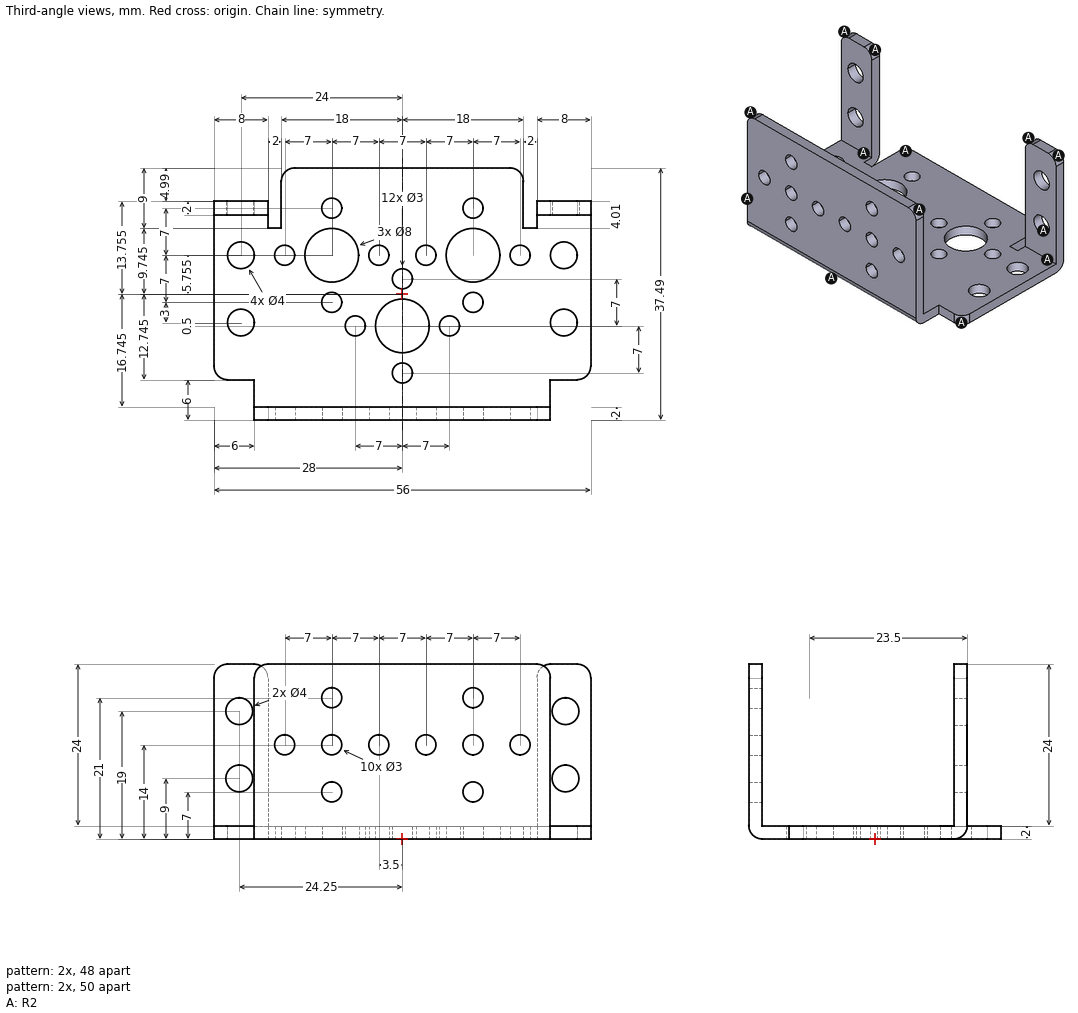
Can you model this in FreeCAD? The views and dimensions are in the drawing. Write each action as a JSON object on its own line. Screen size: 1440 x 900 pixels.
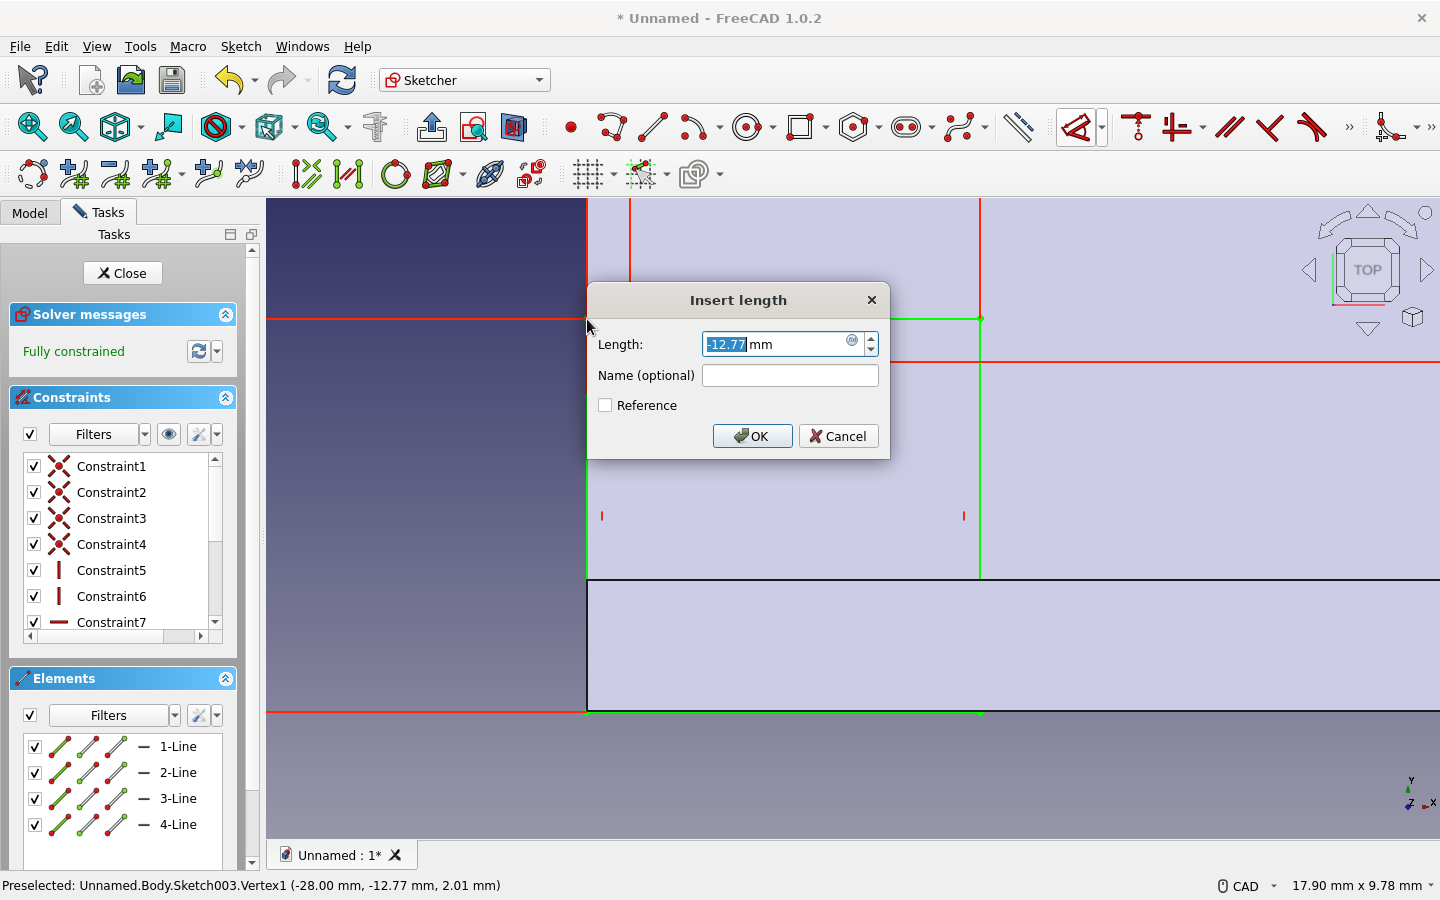
{"action": "type", "text": "-12.745"}
{"action": "key", "text": "Return"}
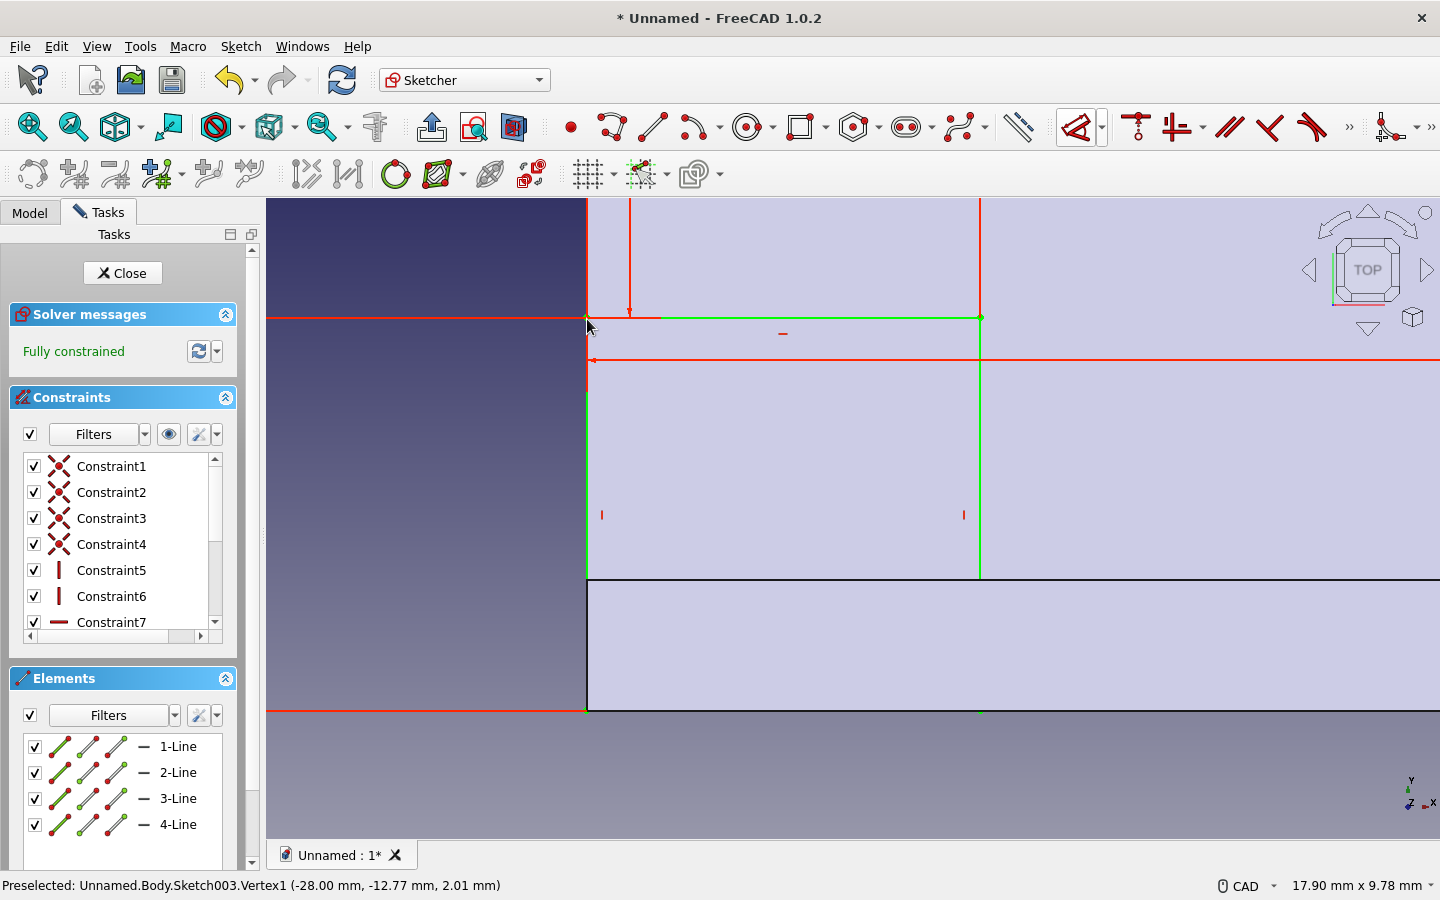
{"action": "left_click", "coordinate": [123, 273]}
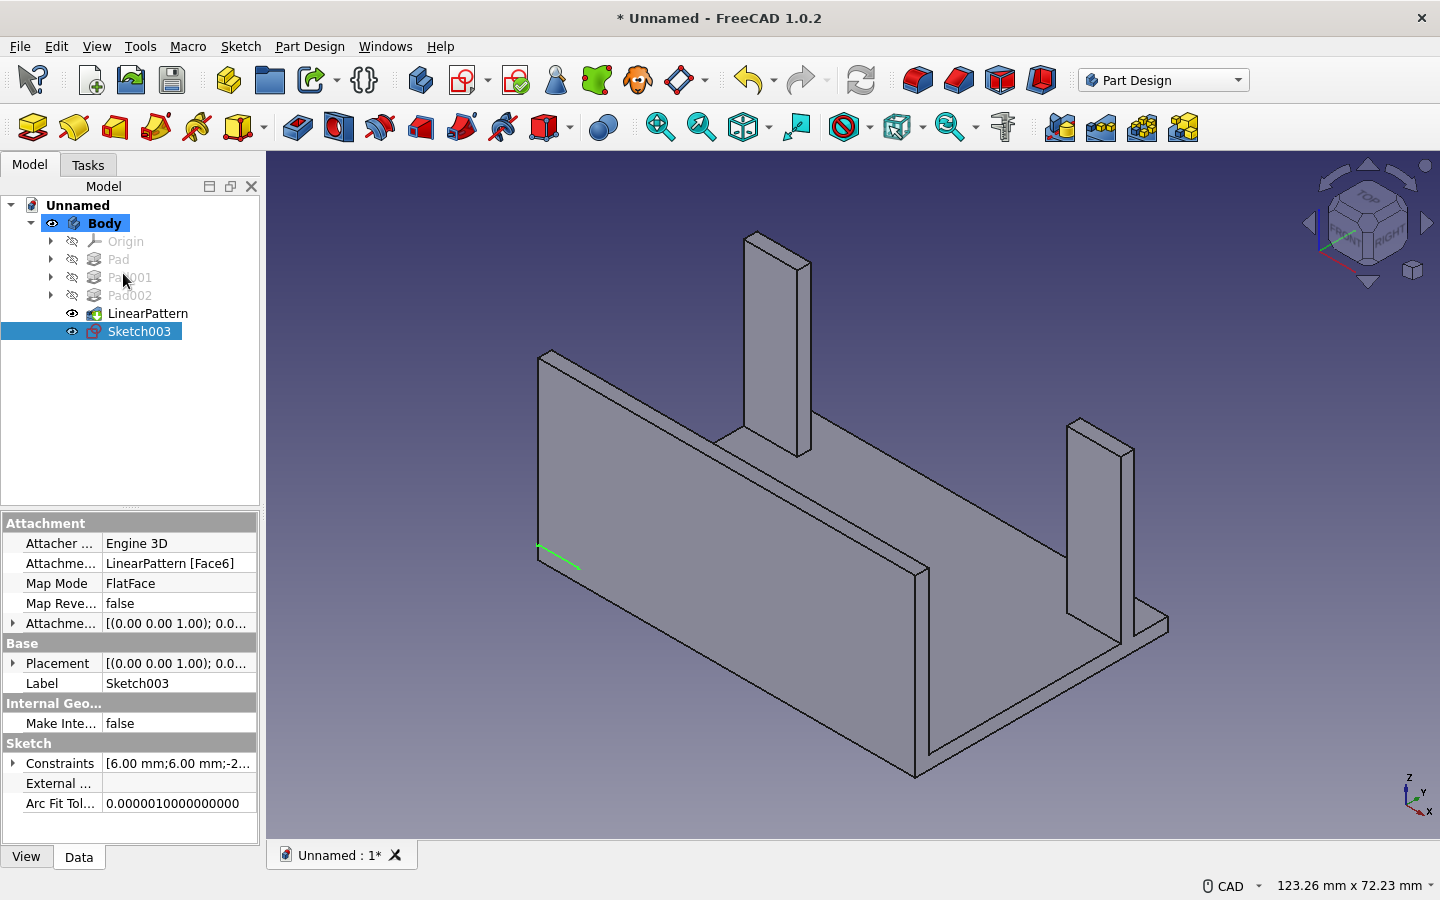
{"action": "left_click", "coordinate": [298, 128]}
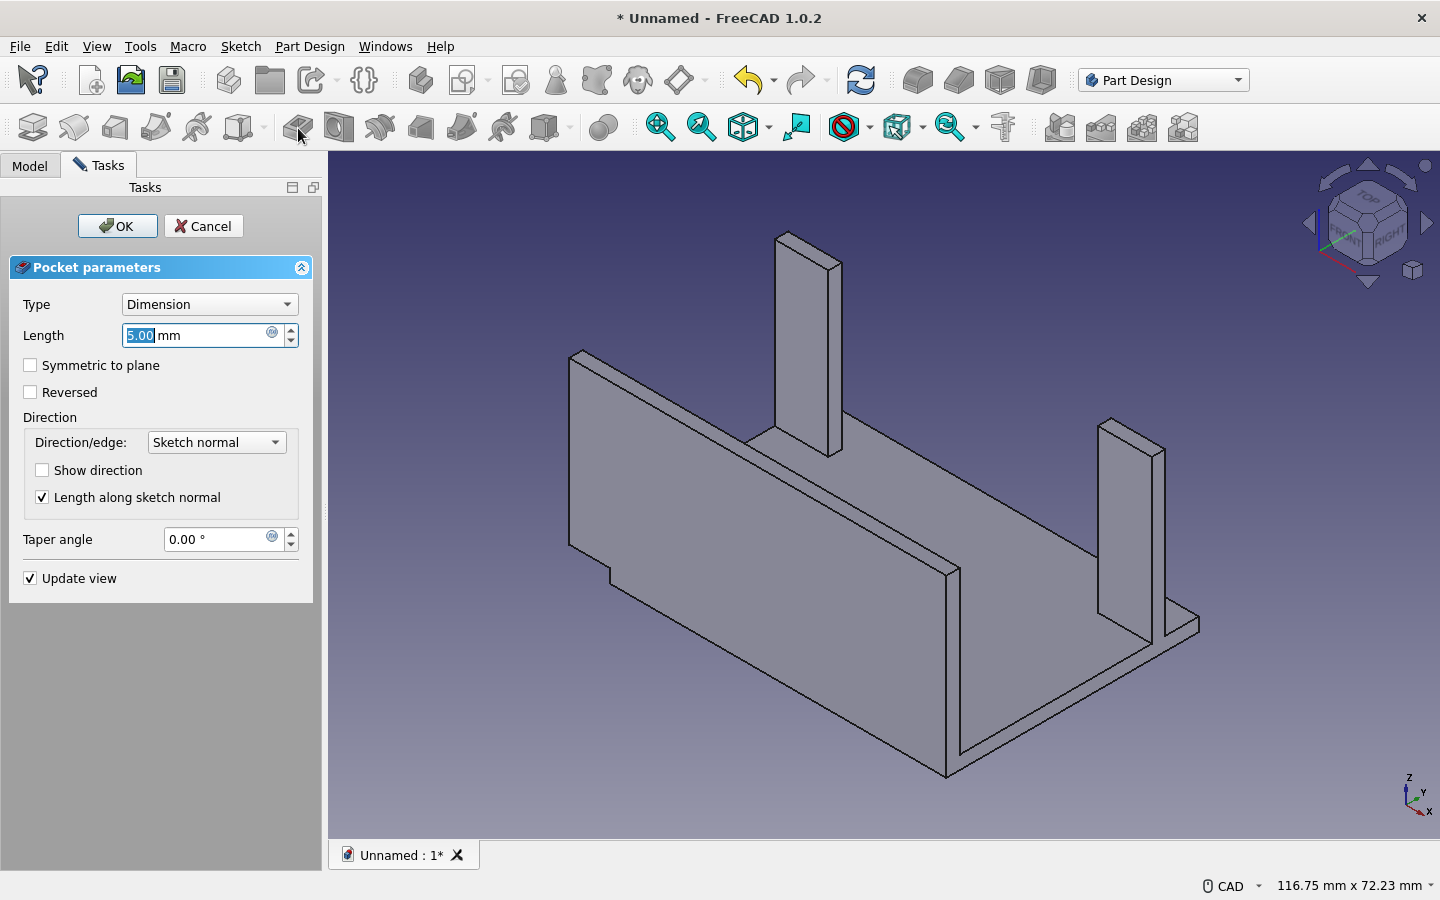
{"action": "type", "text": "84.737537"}
{"action": "key", "text": "Tab"}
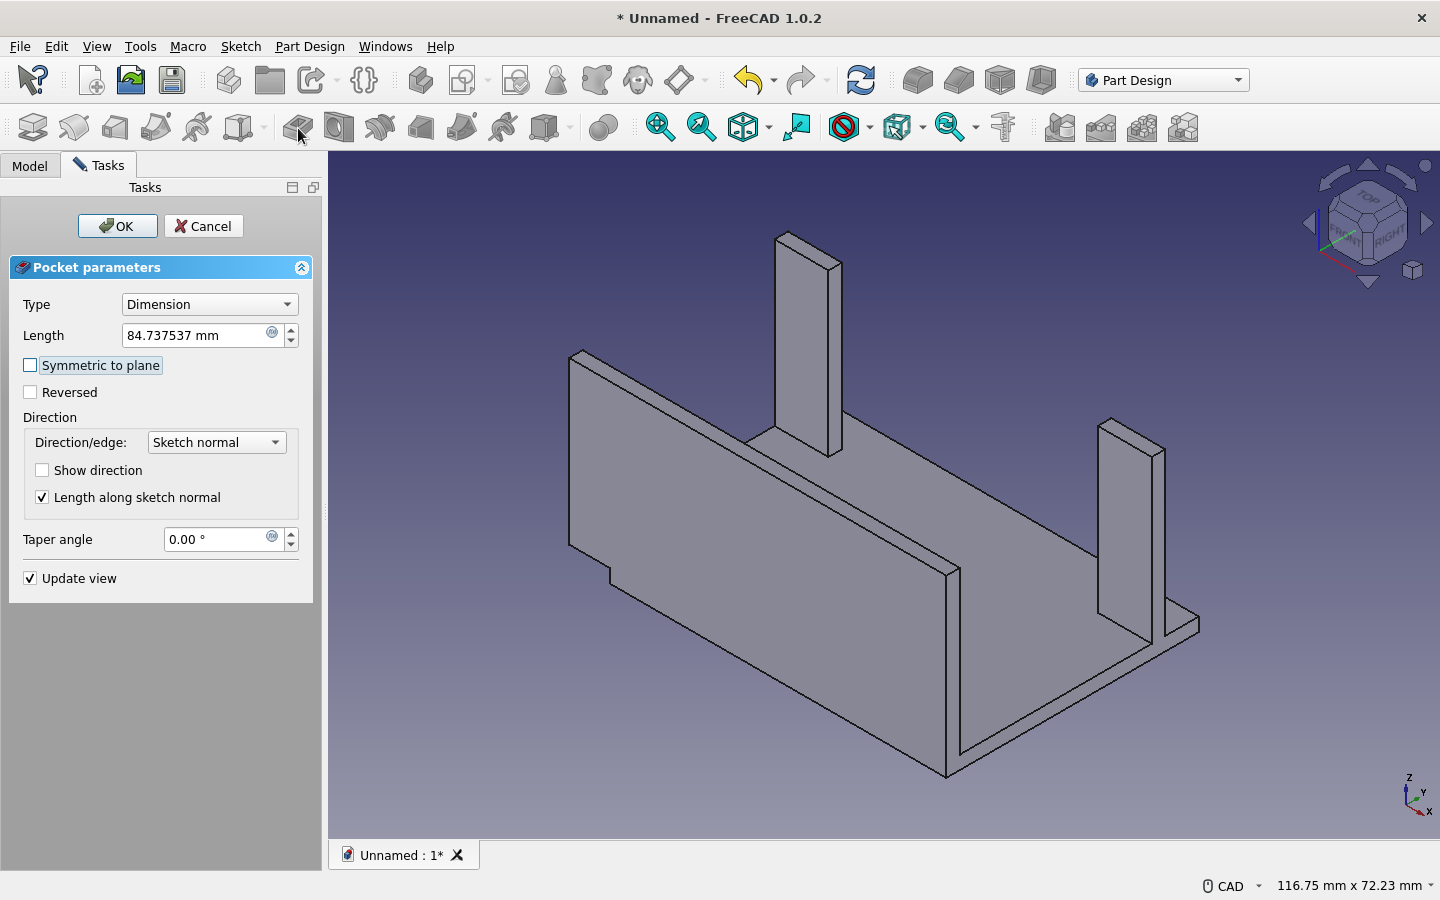
{"action": "left_click", "coordinate": [31, 365]}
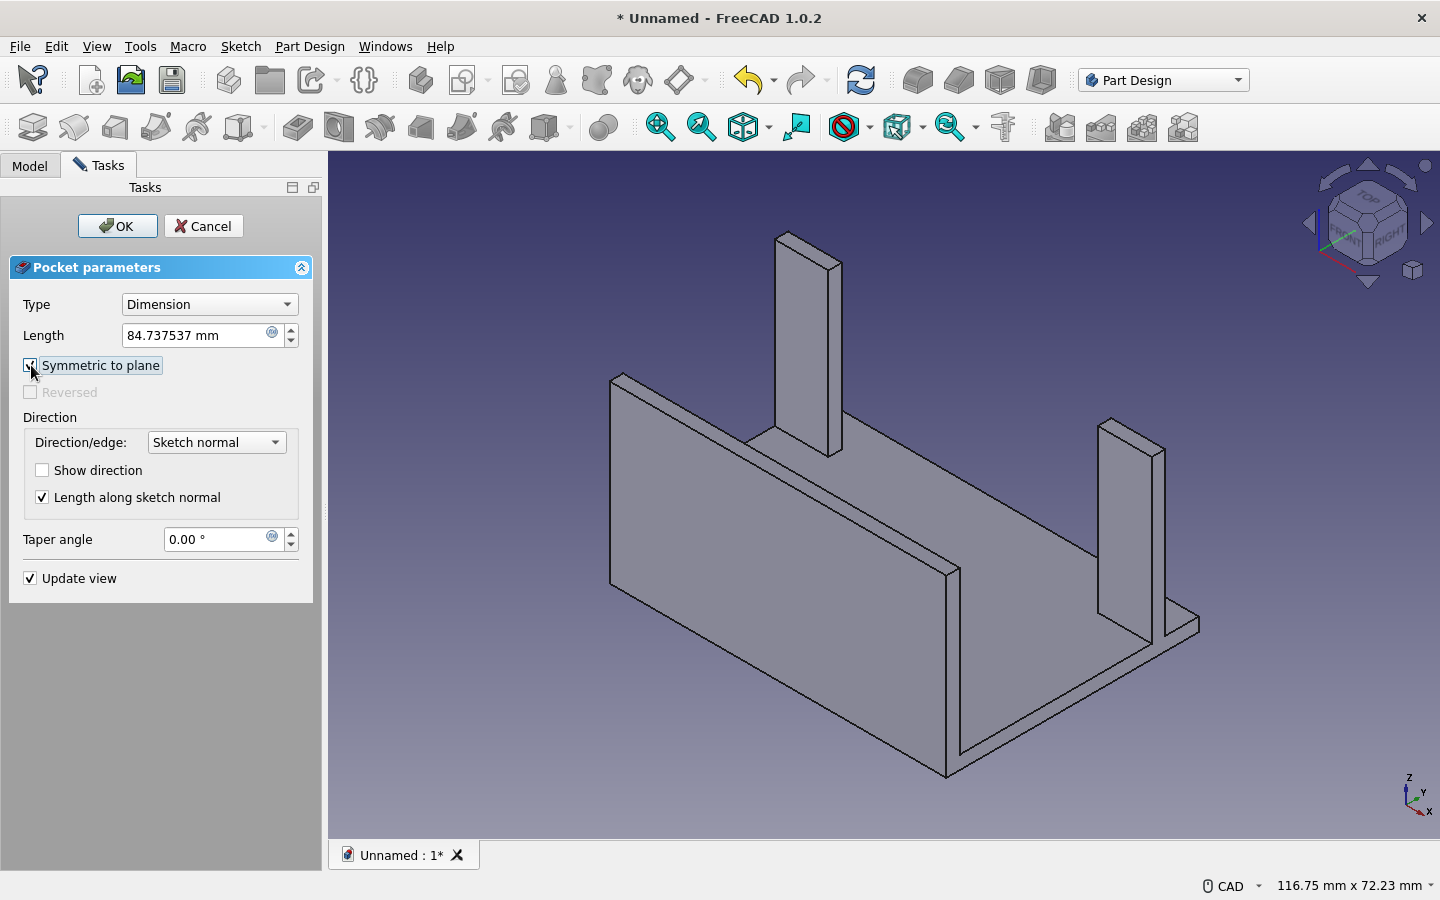
{"action": "left_click", "coordinate": [118, 226]}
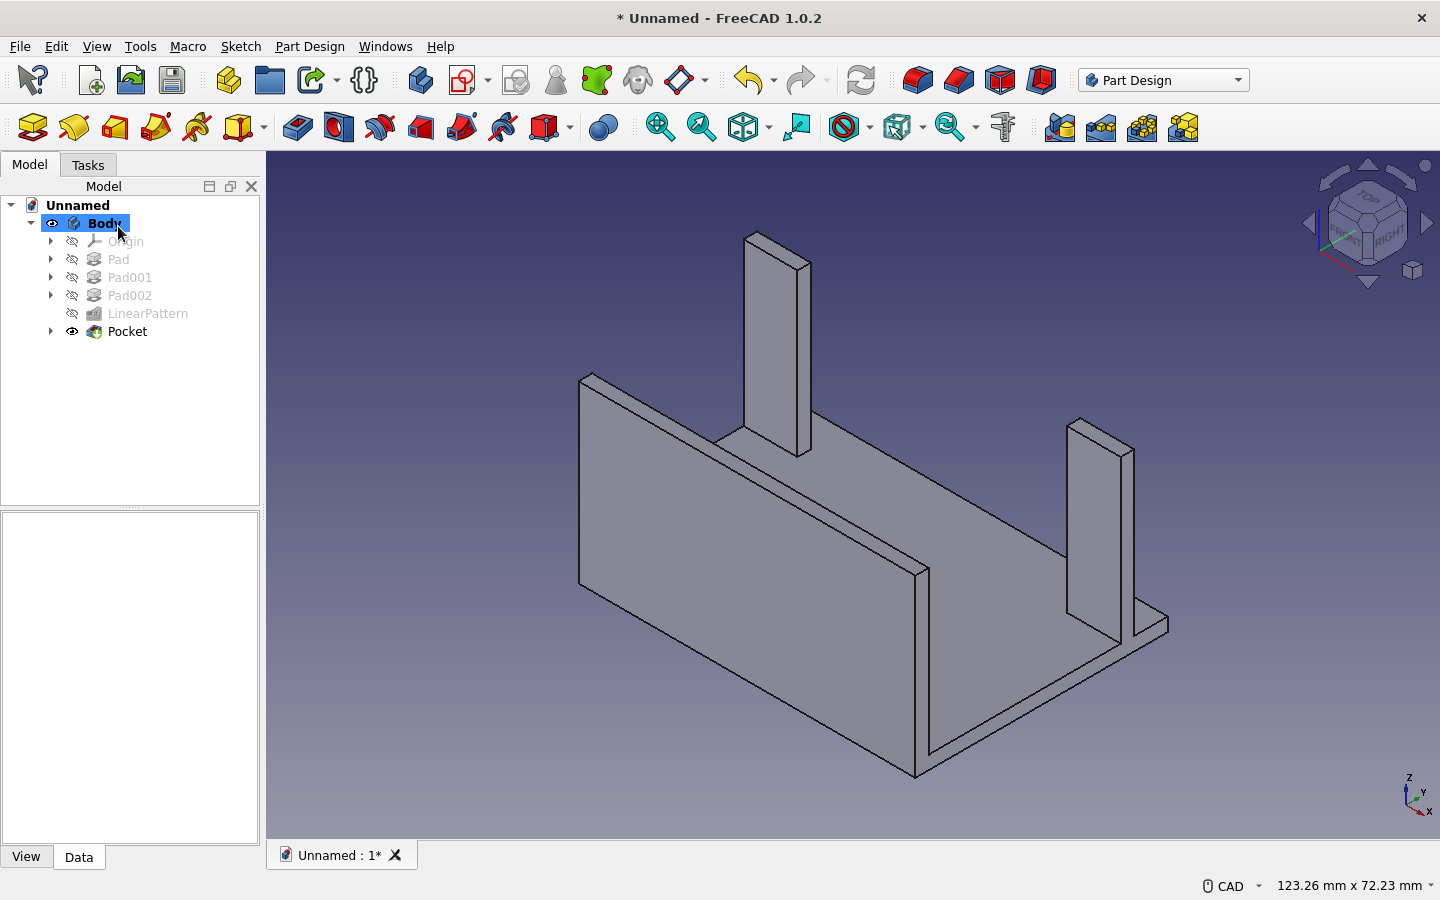
{"action": "left_click", "coordinate": [117, 331]}